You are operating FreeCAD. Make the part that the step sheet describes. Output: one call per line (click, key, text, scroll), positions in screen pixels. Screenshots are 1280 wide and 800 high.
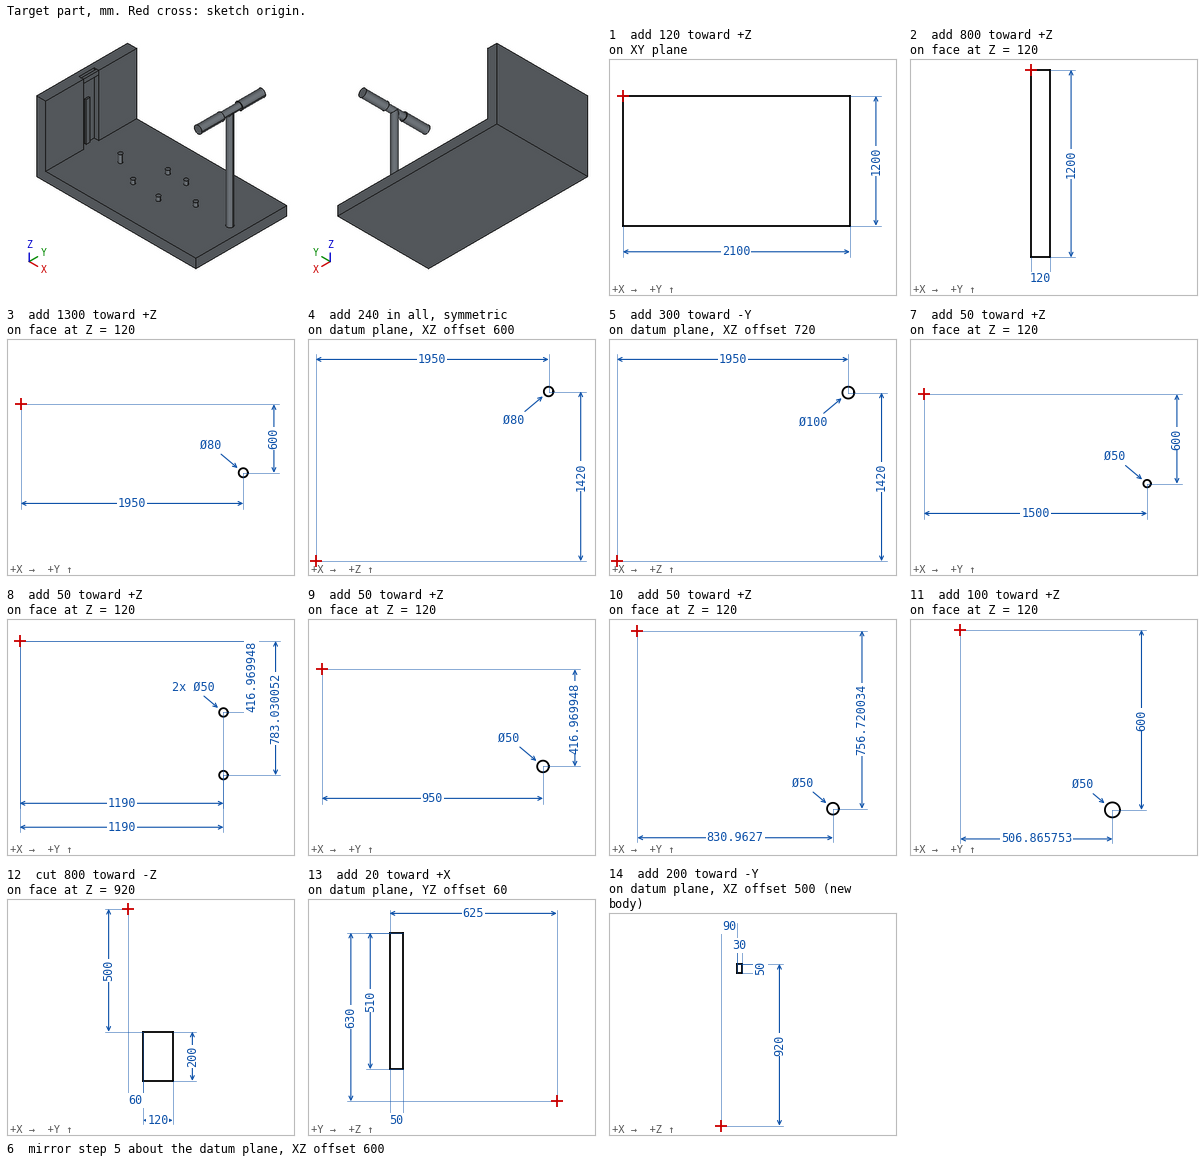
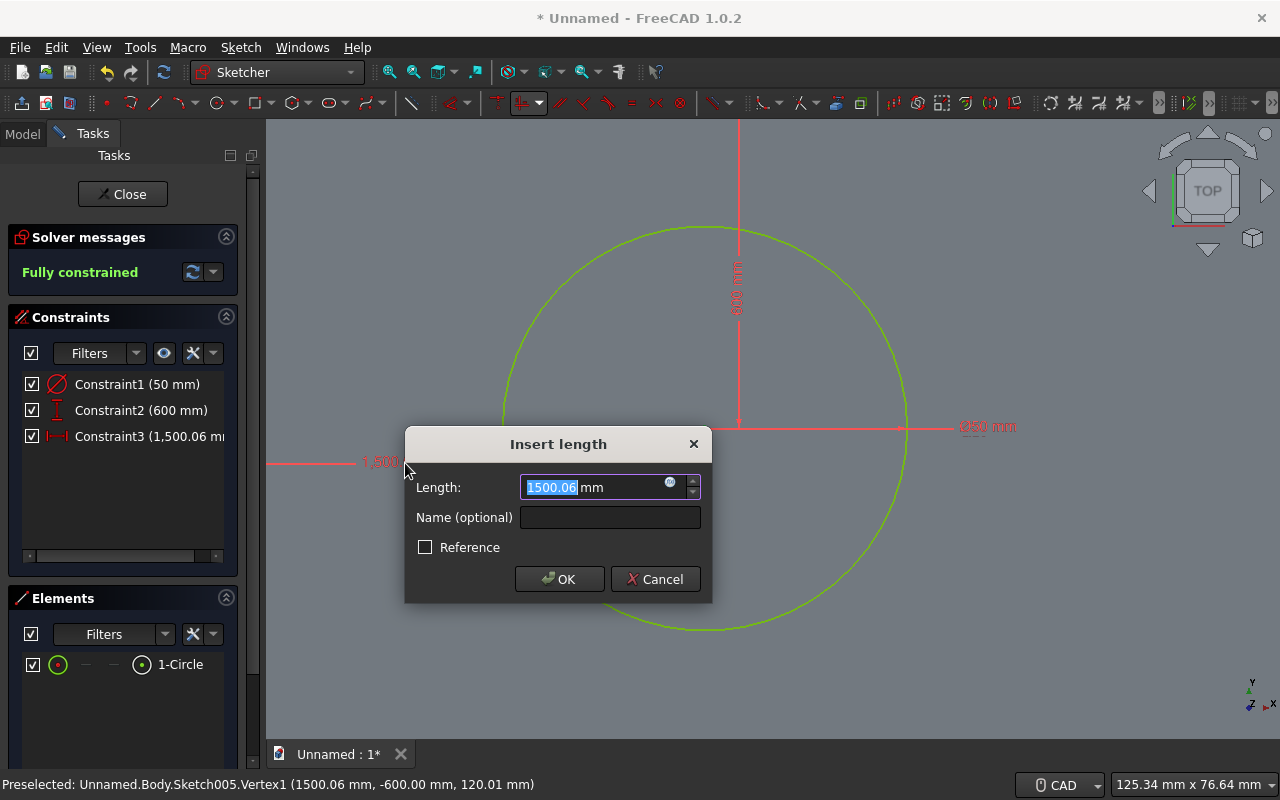
text(1500)
key(Return)
key(Escape)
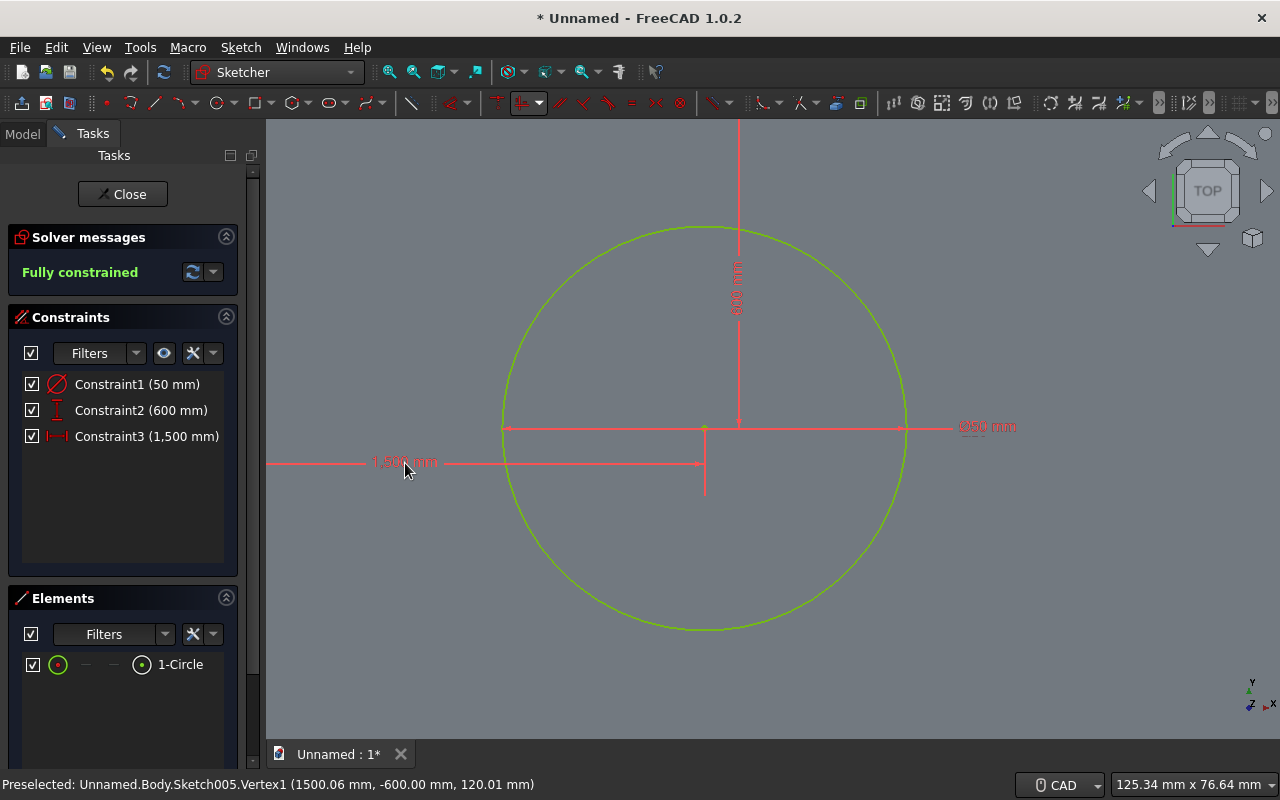
click(123, 194)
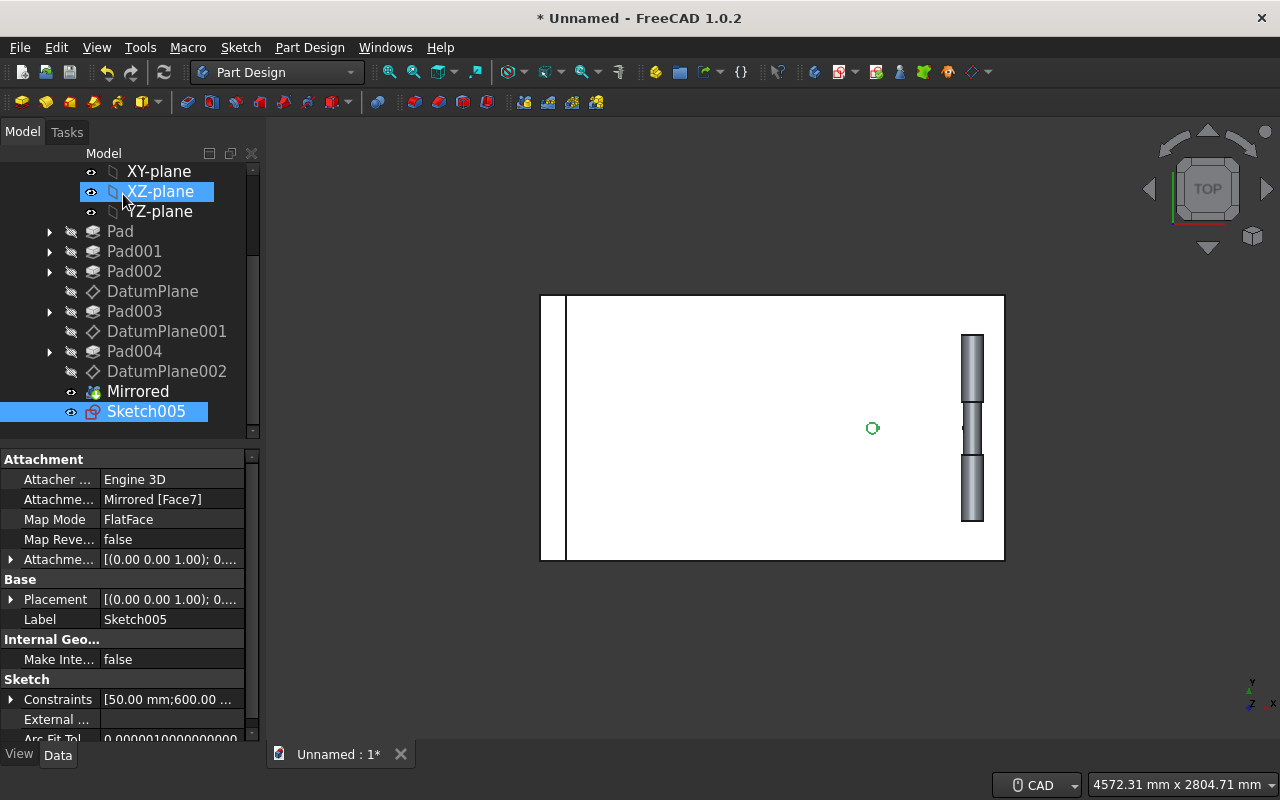
click(22, 102)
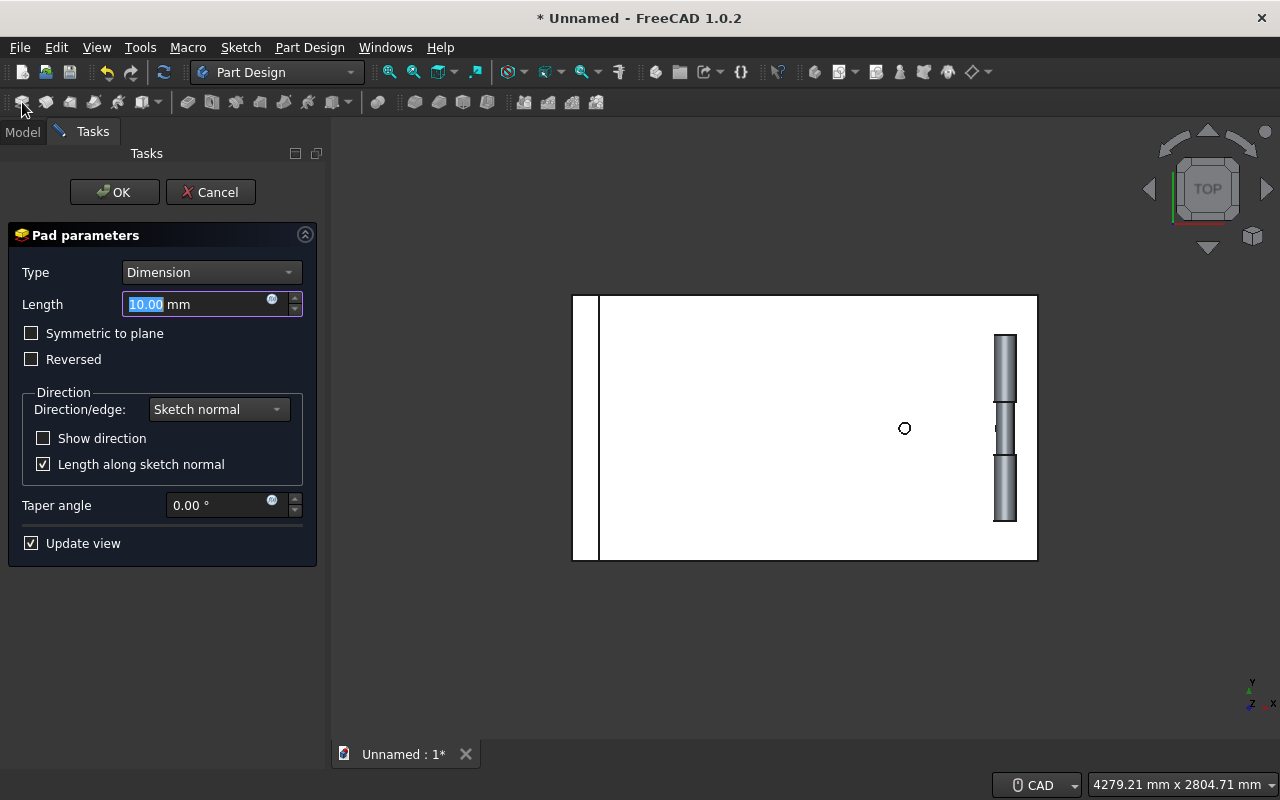
text(50)
key(Tab)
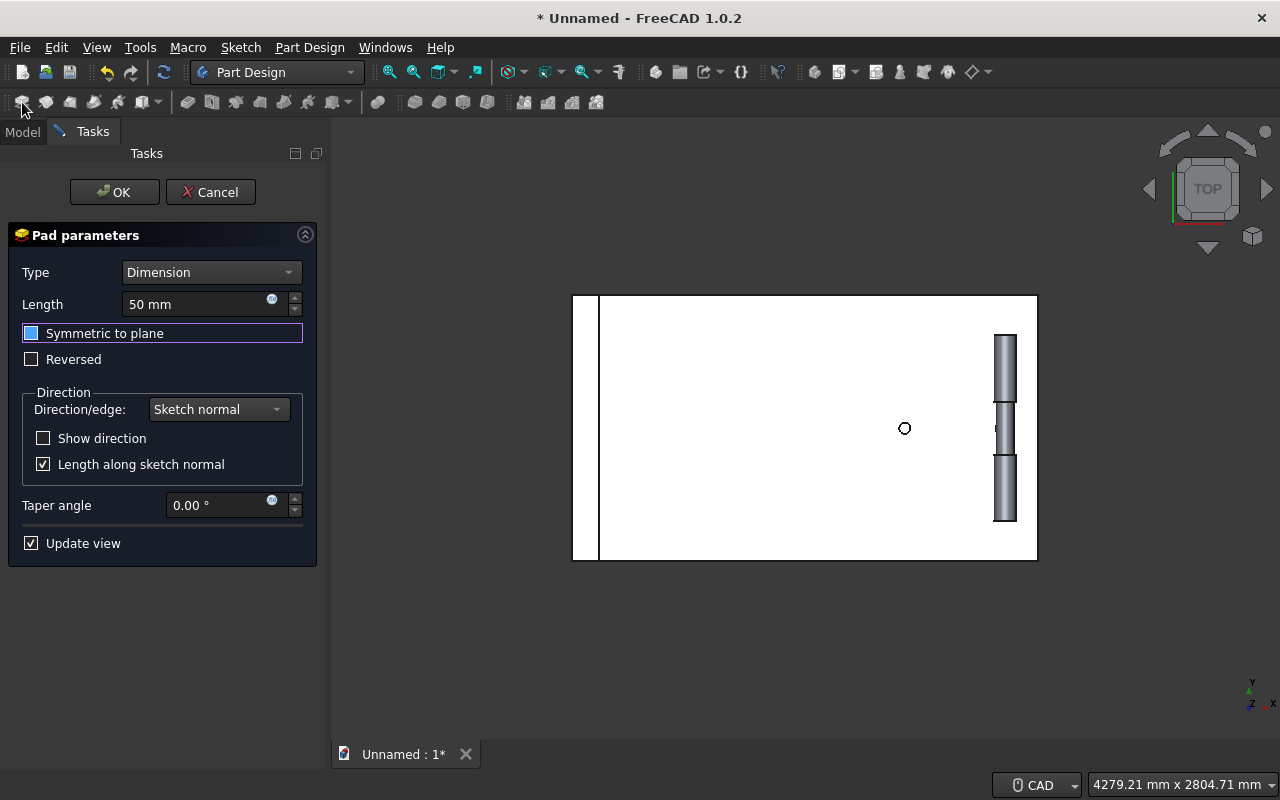
click(115, 192)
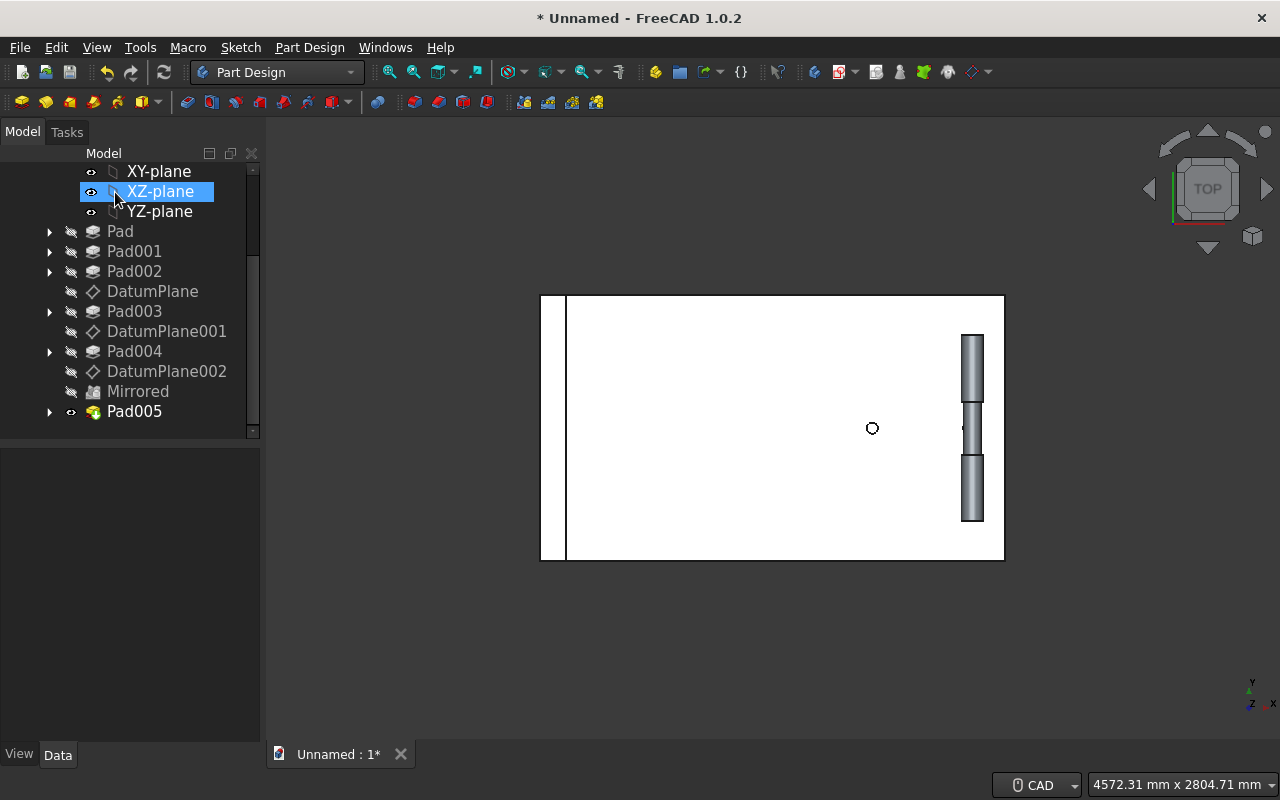
click(723, 427)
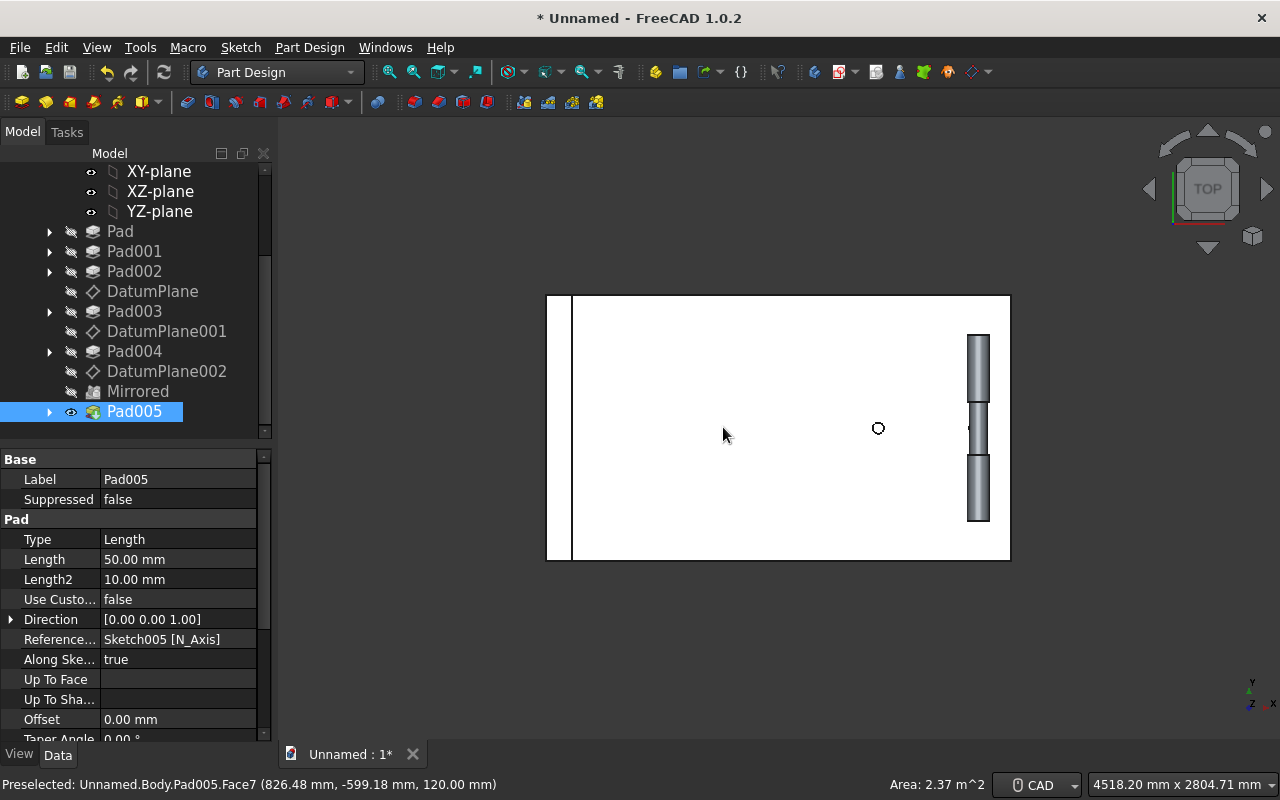
click(840, 72)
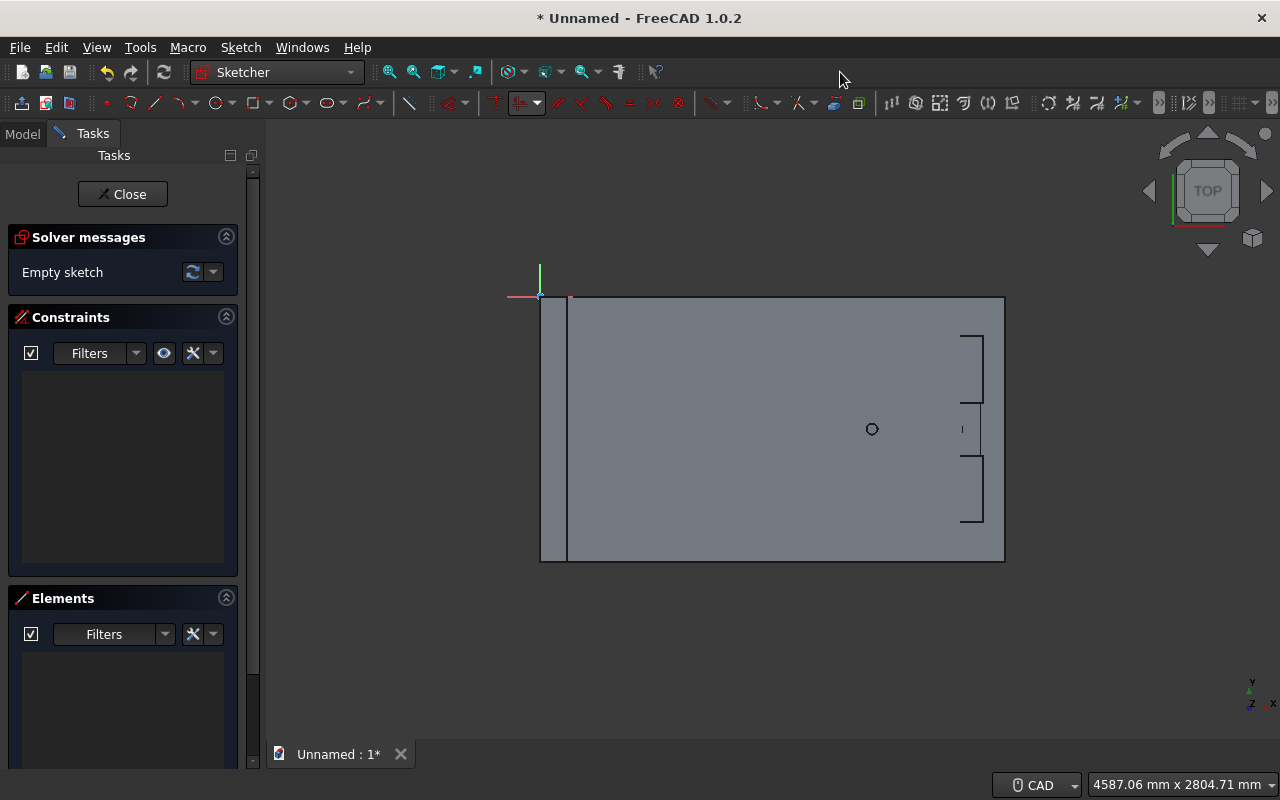
scroll(836, 429, up, 7)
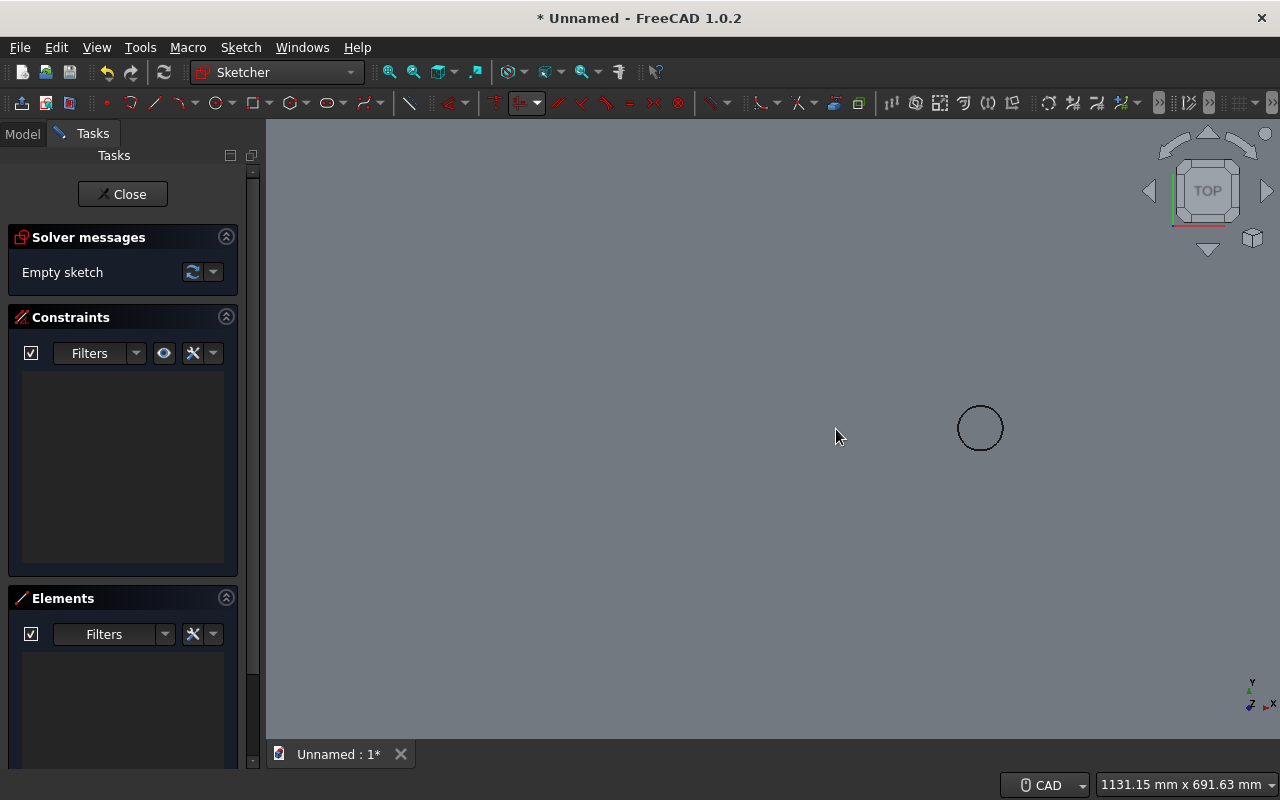
click(216, 104)